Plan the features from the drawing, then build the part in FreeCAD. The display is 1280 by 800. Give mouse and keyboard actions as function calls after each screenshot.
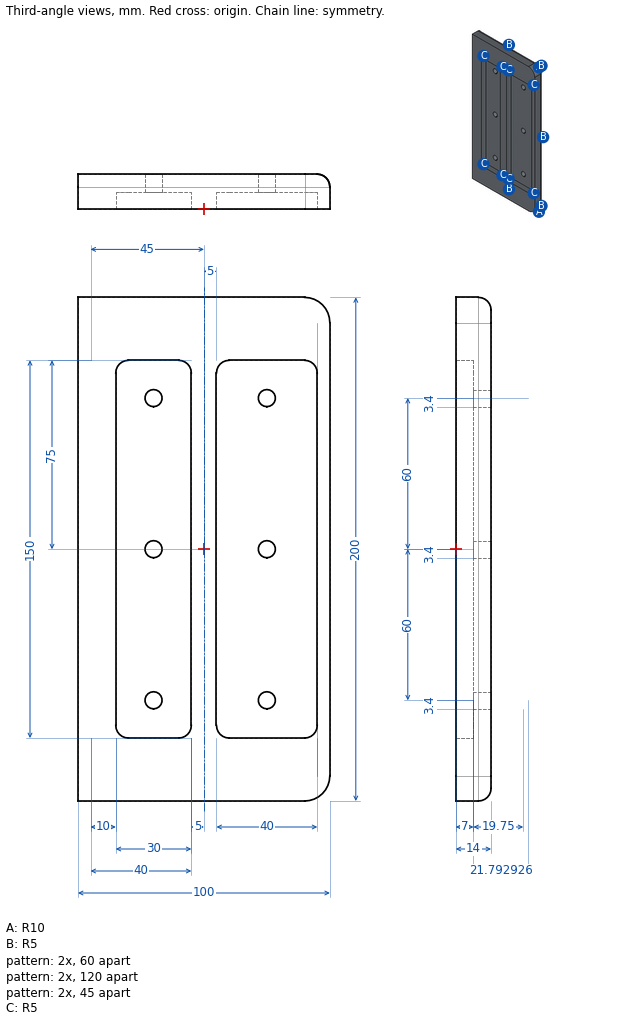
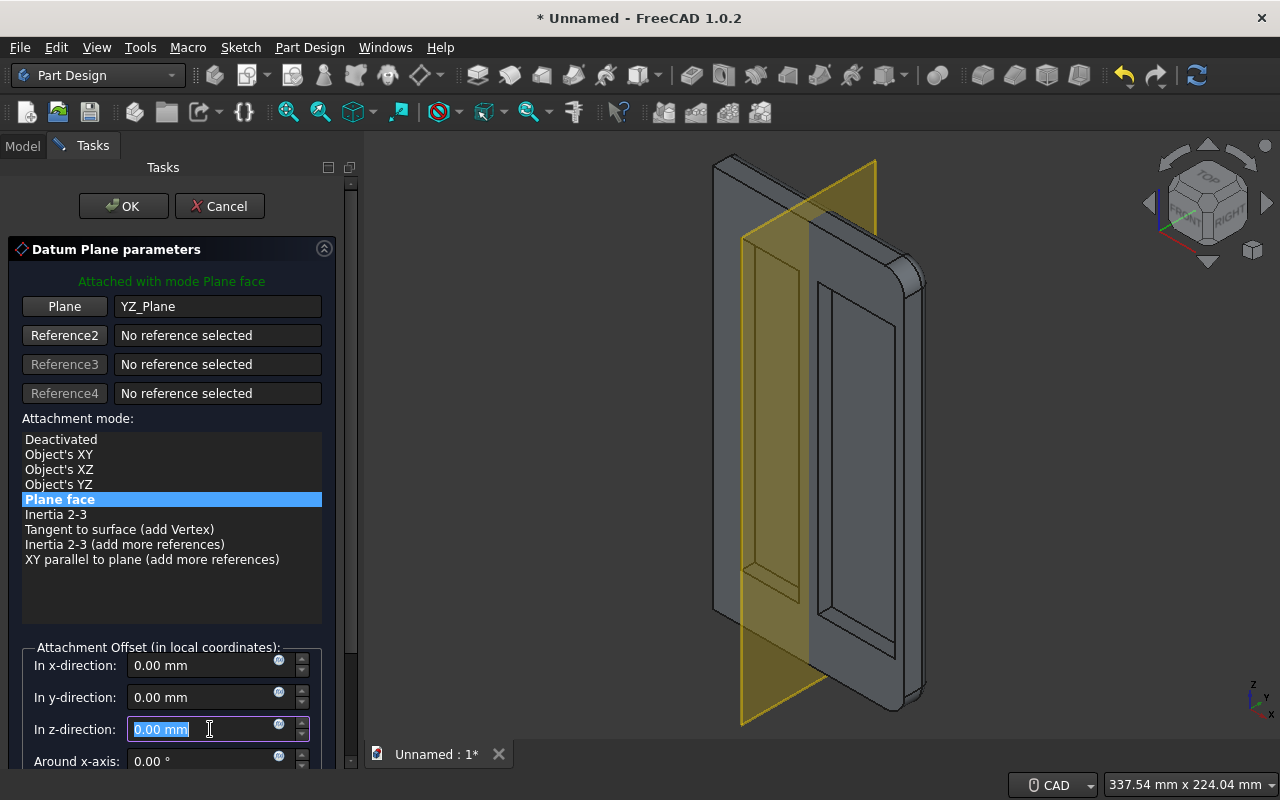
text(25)
key(Tab)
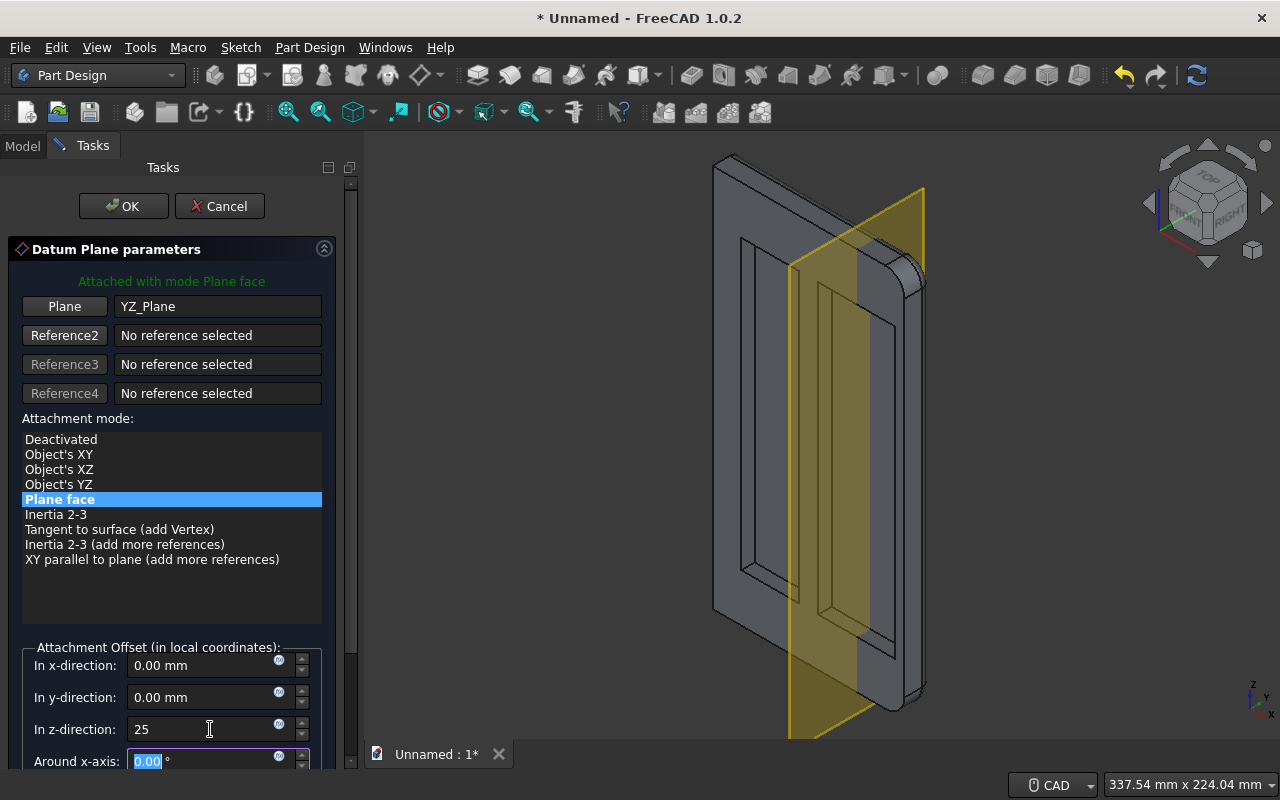
click(124, 206)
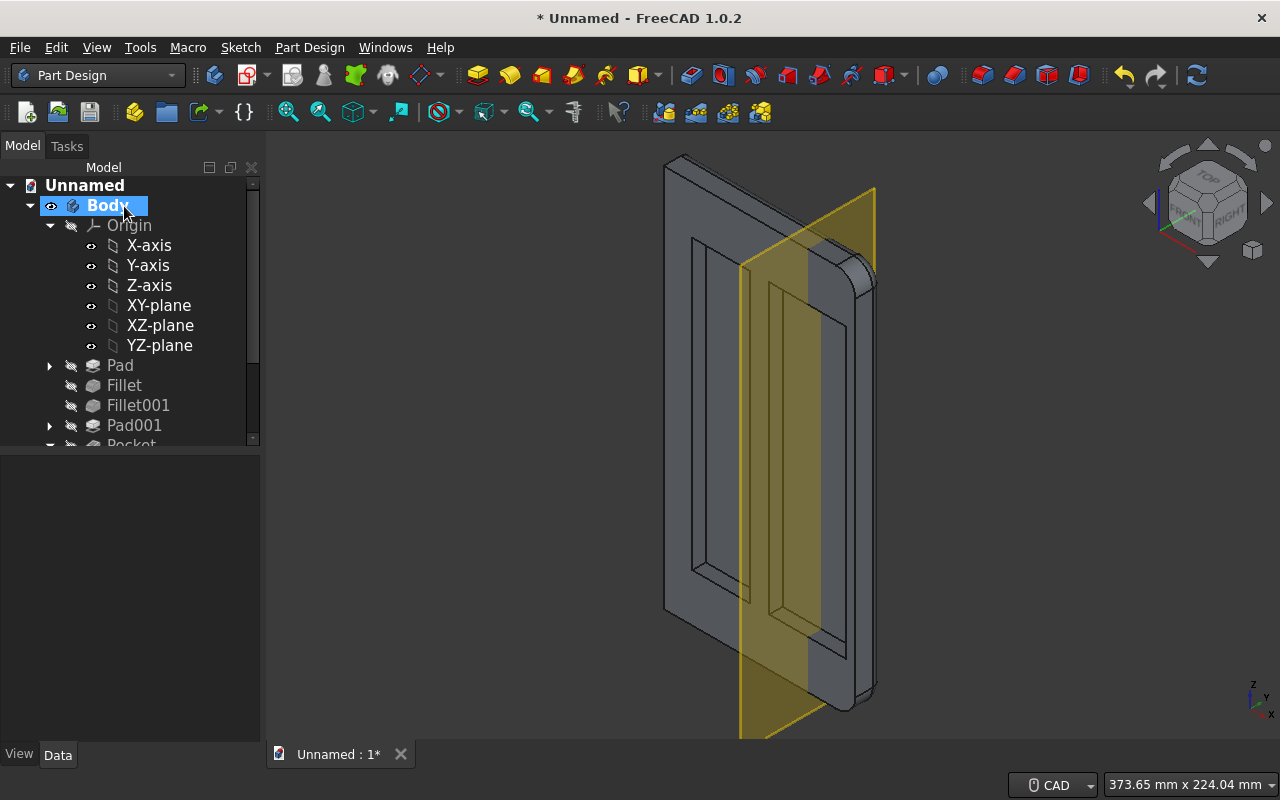
scroll(100, 321, down, 3)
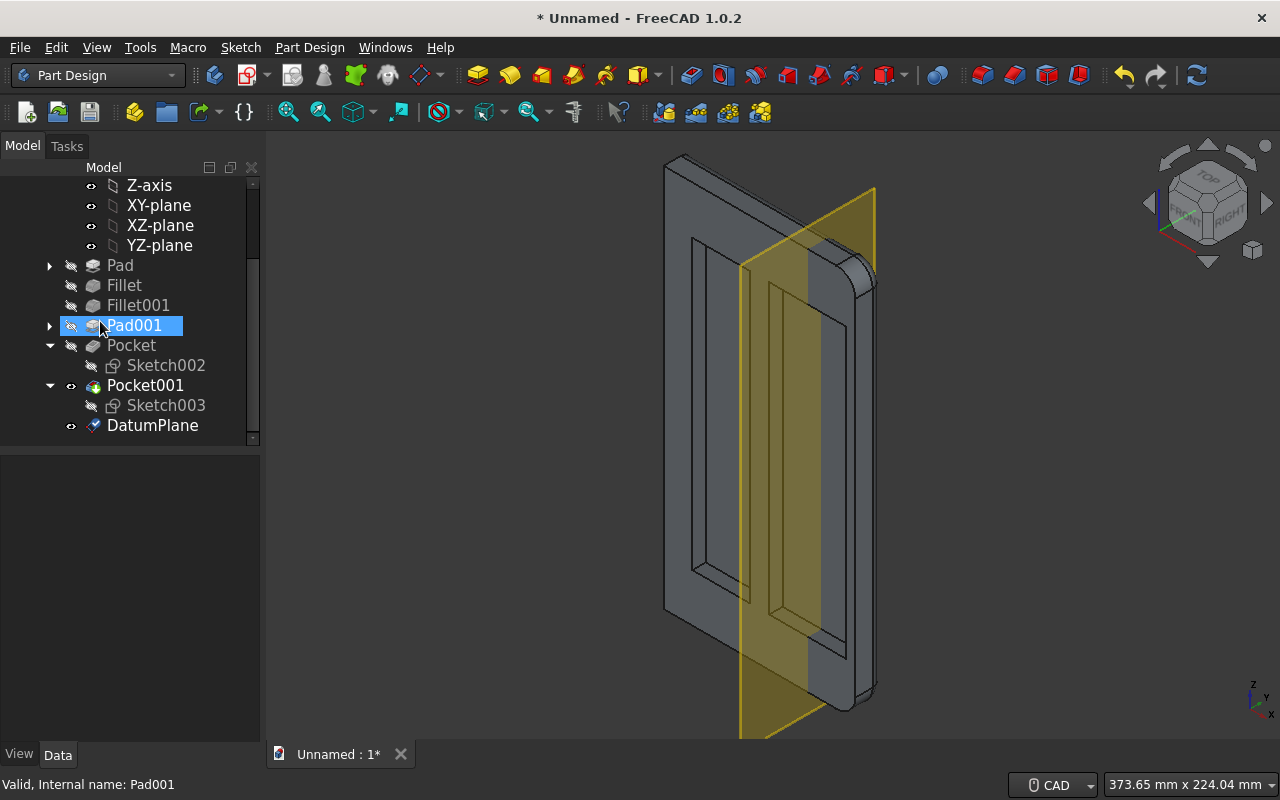
click(116, 426)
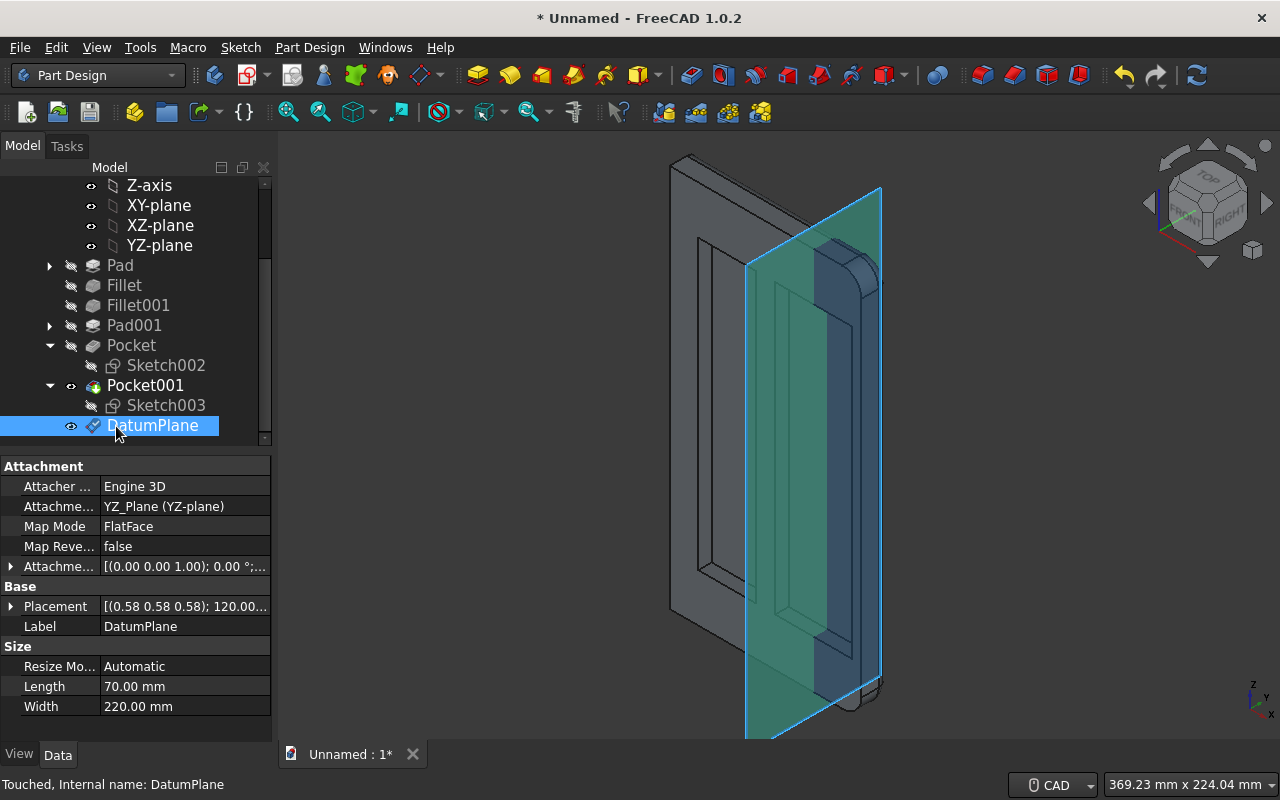
click(248, 76)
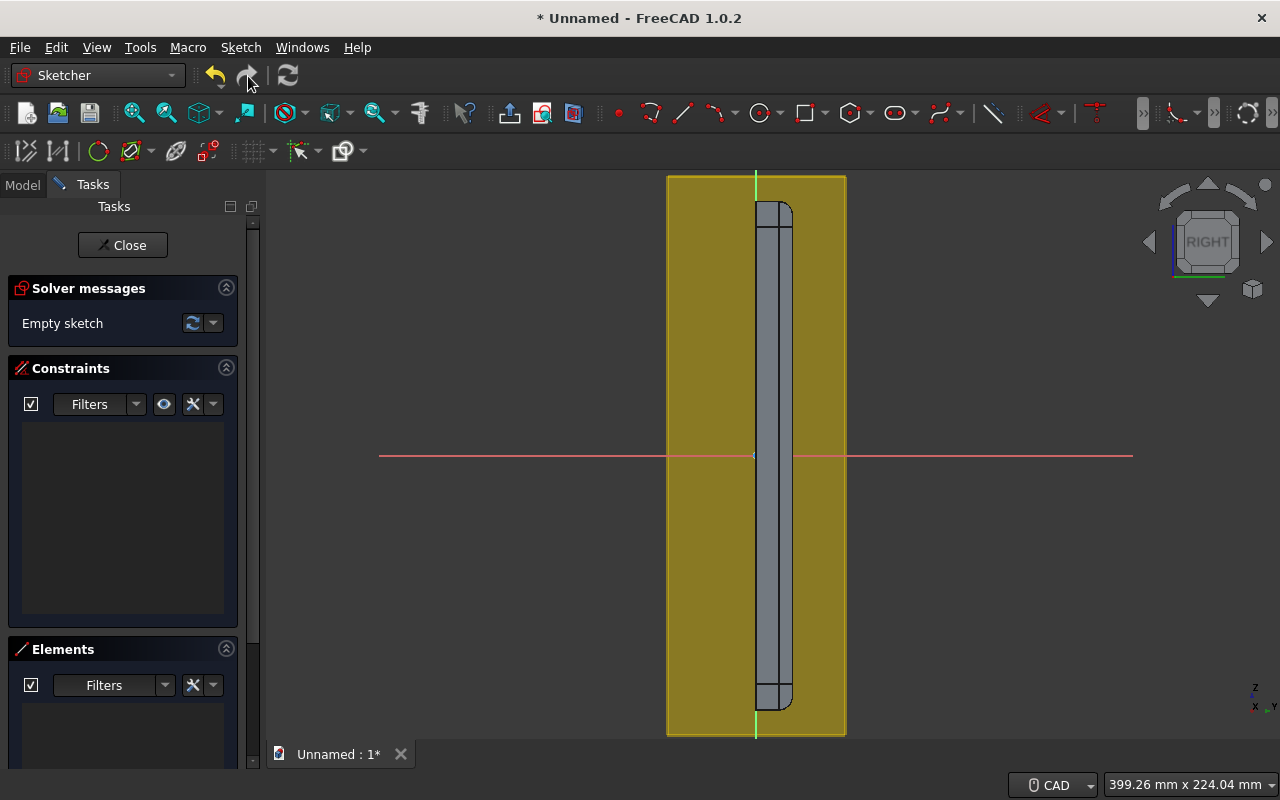
key(q)
key(s)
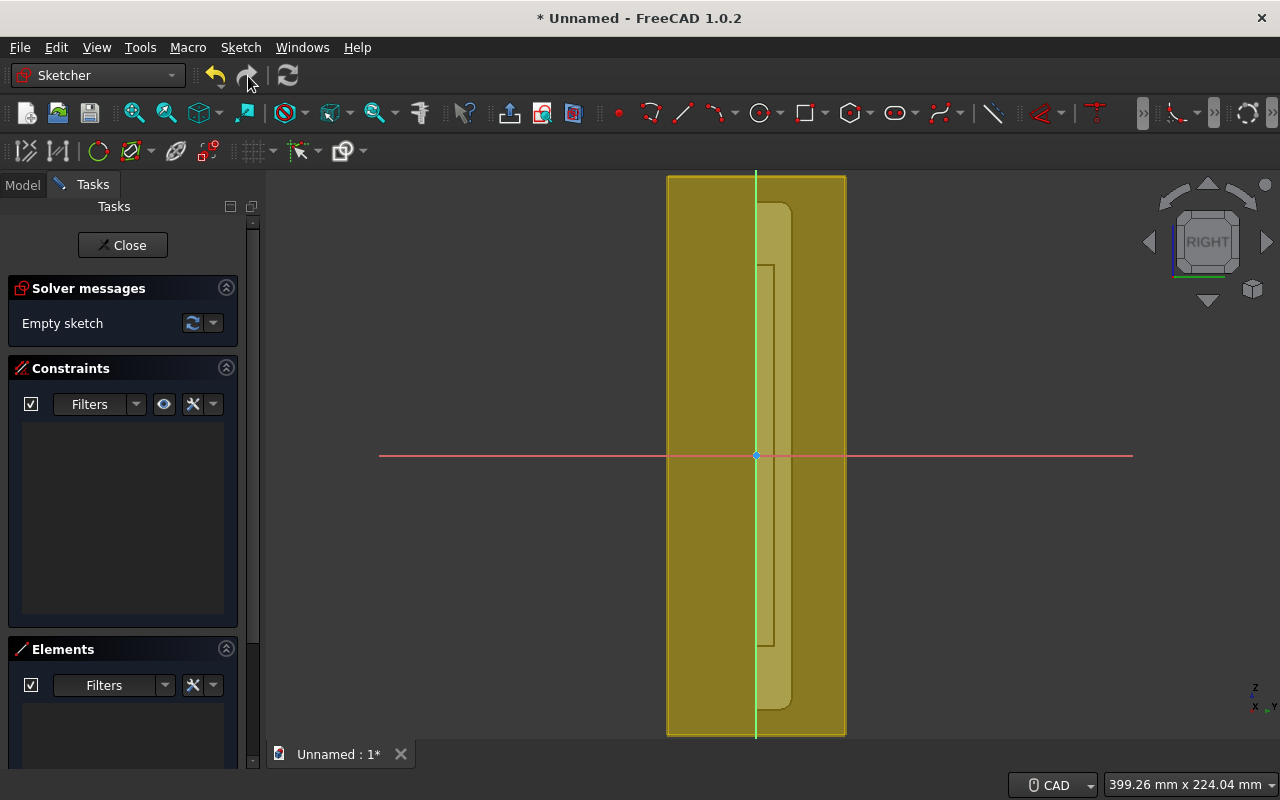
scroll(885, 603, up, 4)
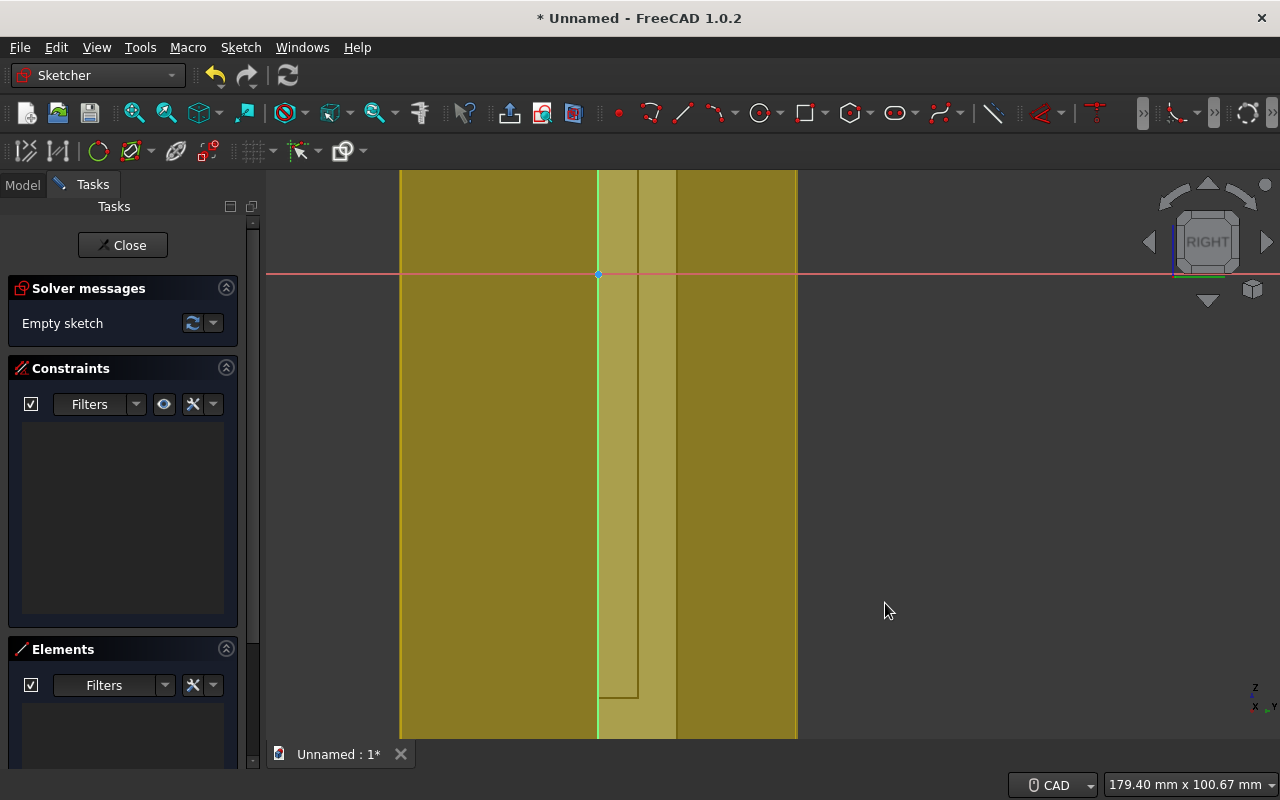
click(652, 114)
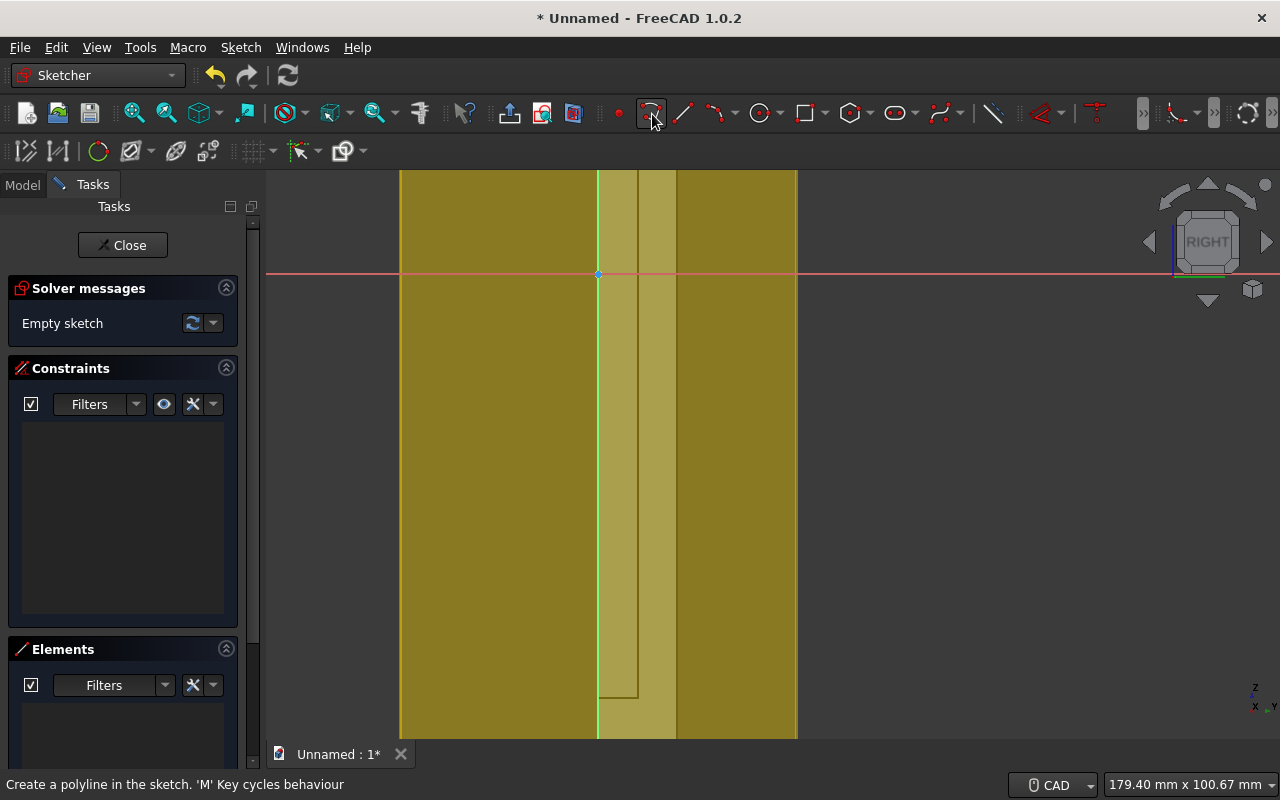
click(638, 614)
click(638, 633)
click(749, 633)
click(761, 614)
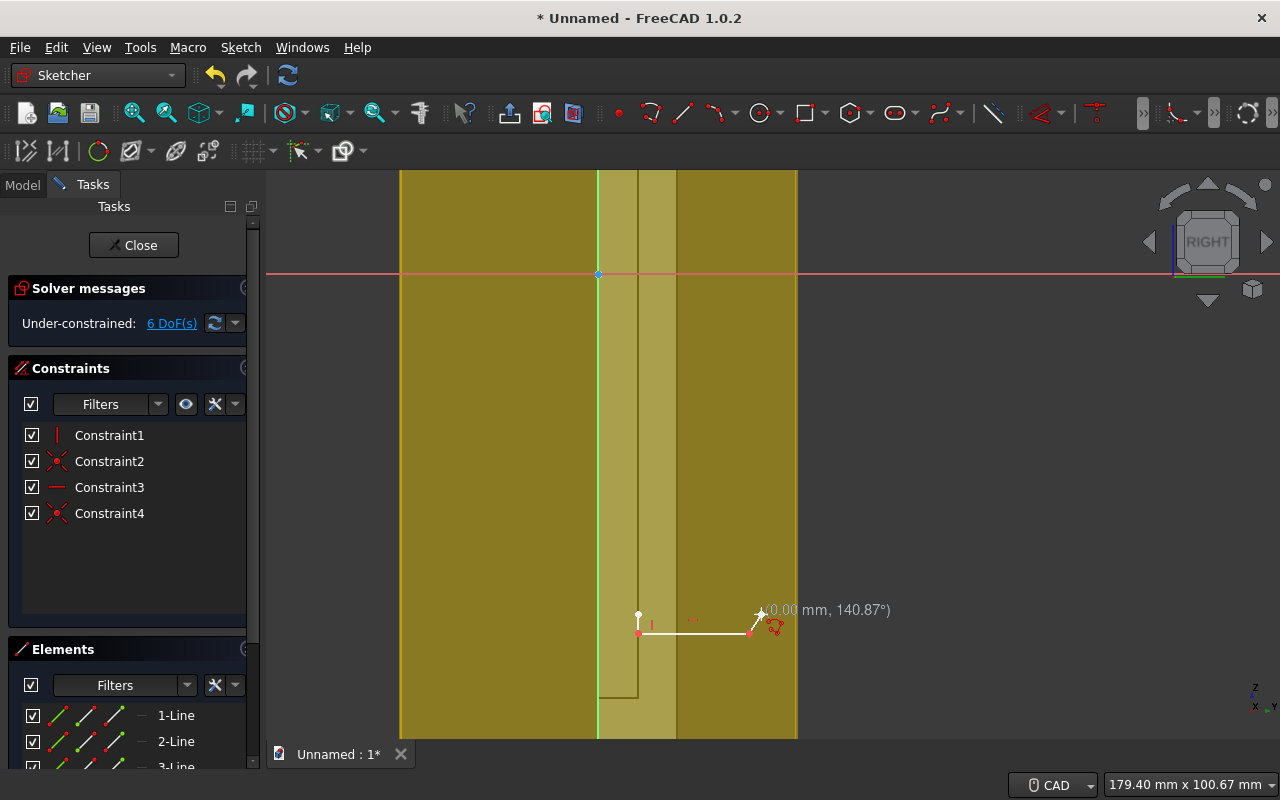
scroll(638, 614, up, 3)